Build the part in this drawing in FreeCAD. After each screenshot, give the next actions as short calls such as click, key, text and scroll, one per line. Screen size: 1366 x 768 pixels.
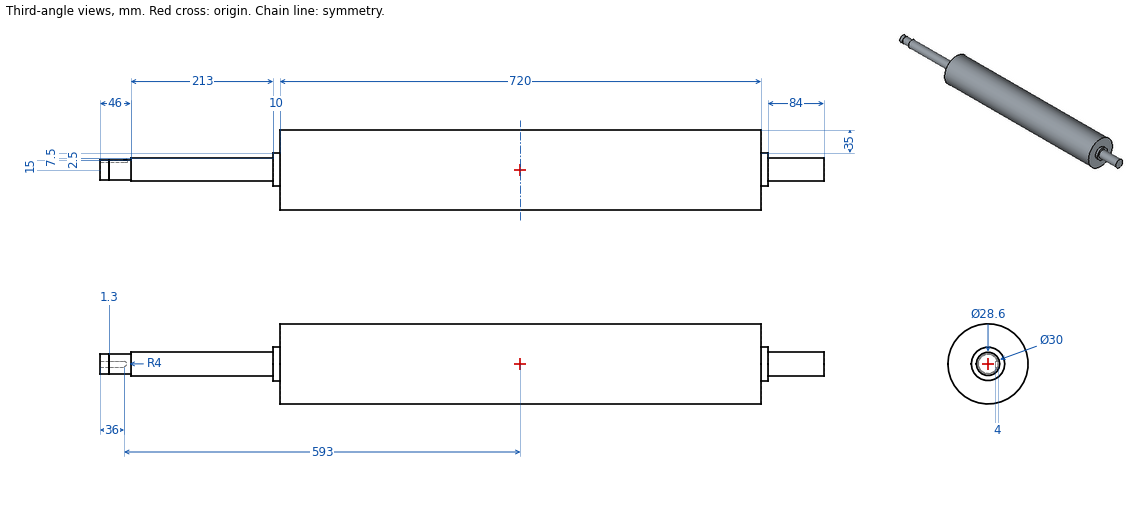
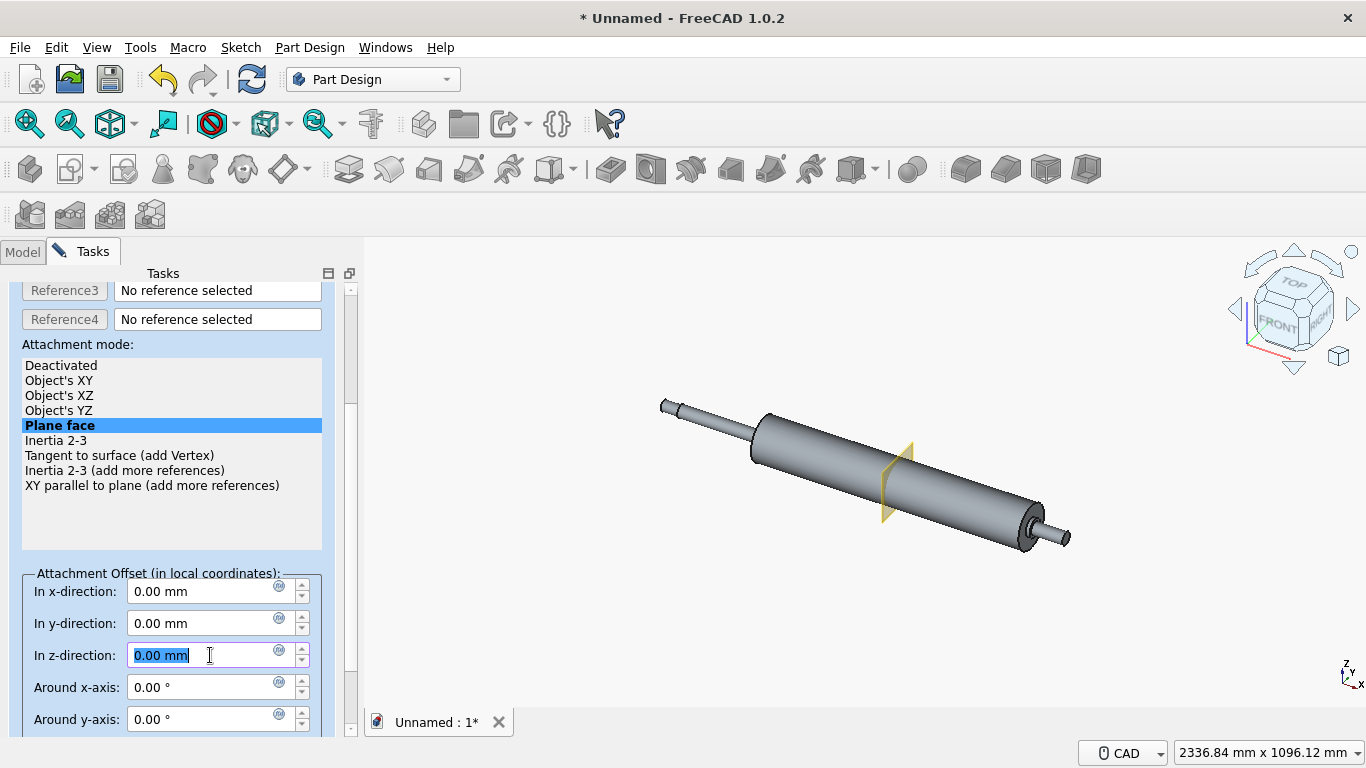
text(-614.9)
key(Tab)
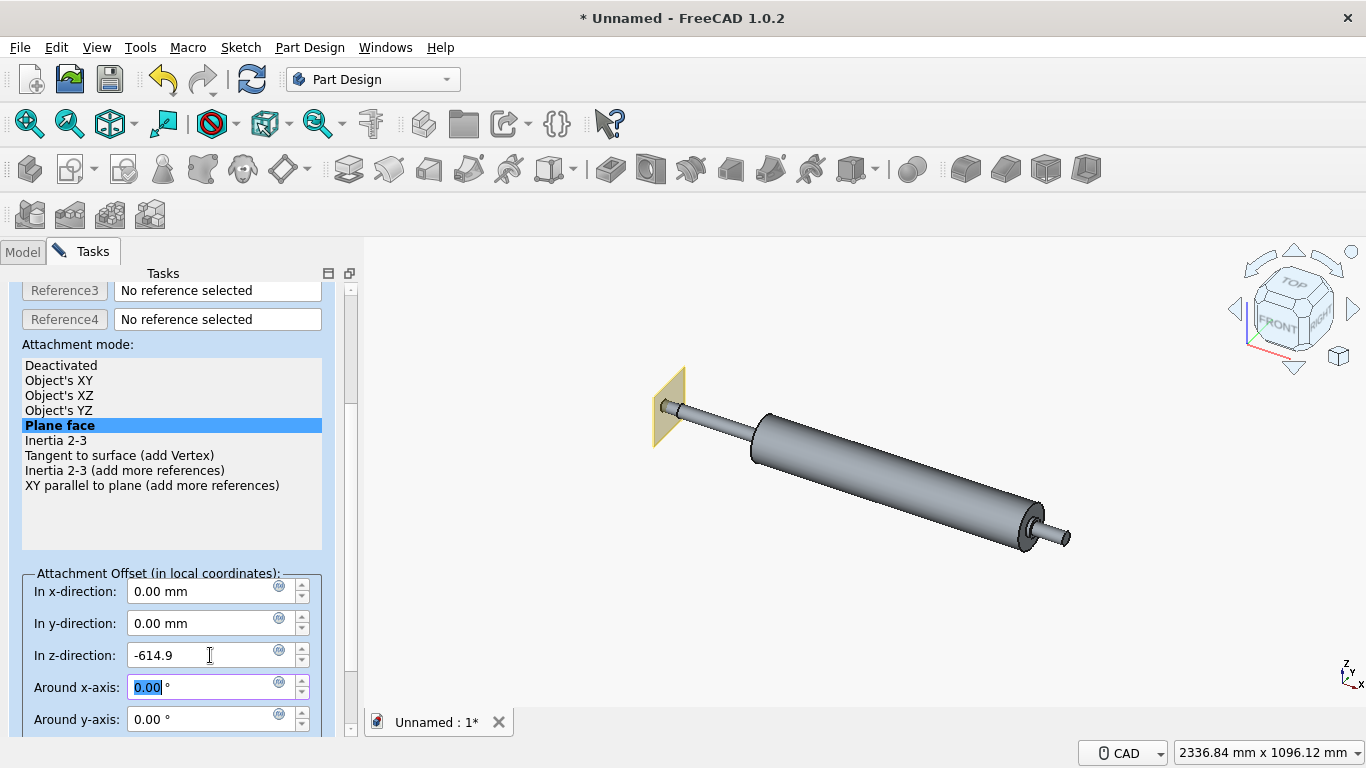
scroll(351, 510, up, 4)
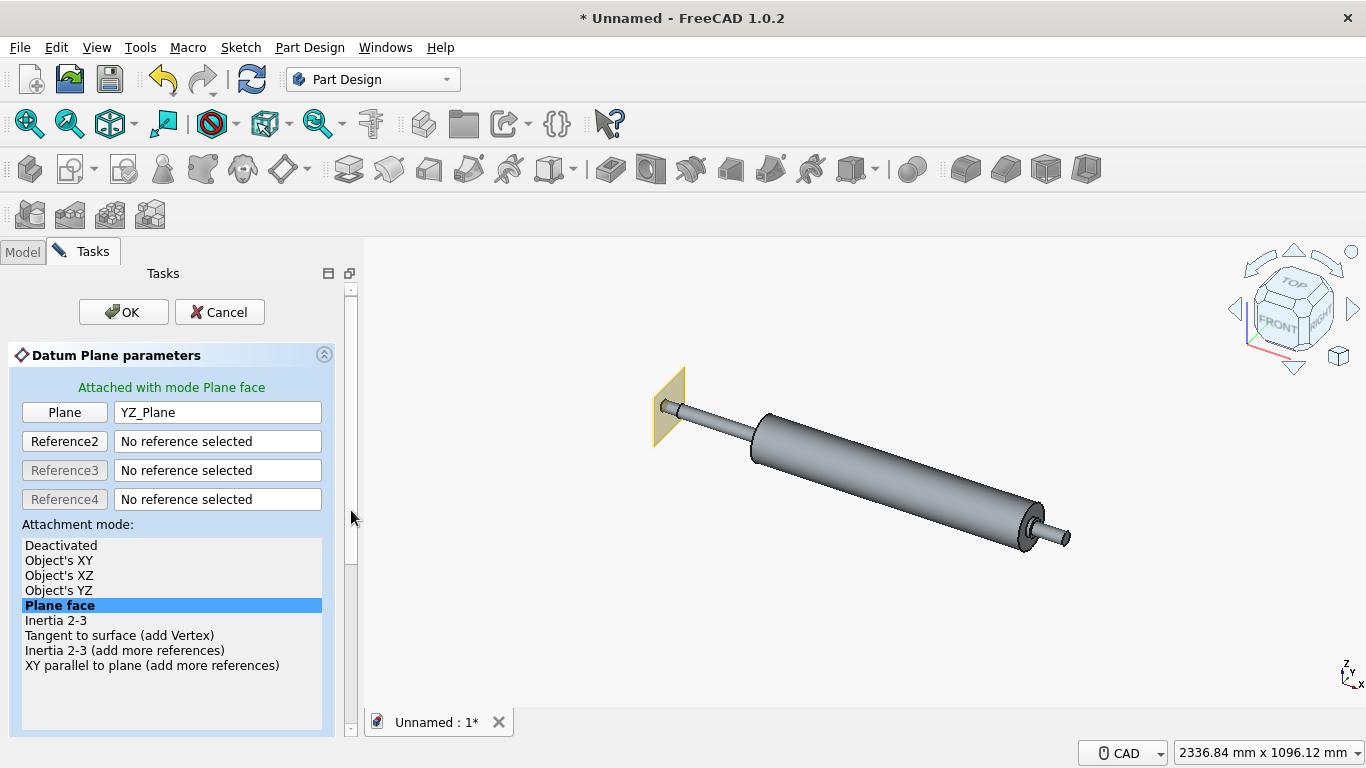
click(124, 312)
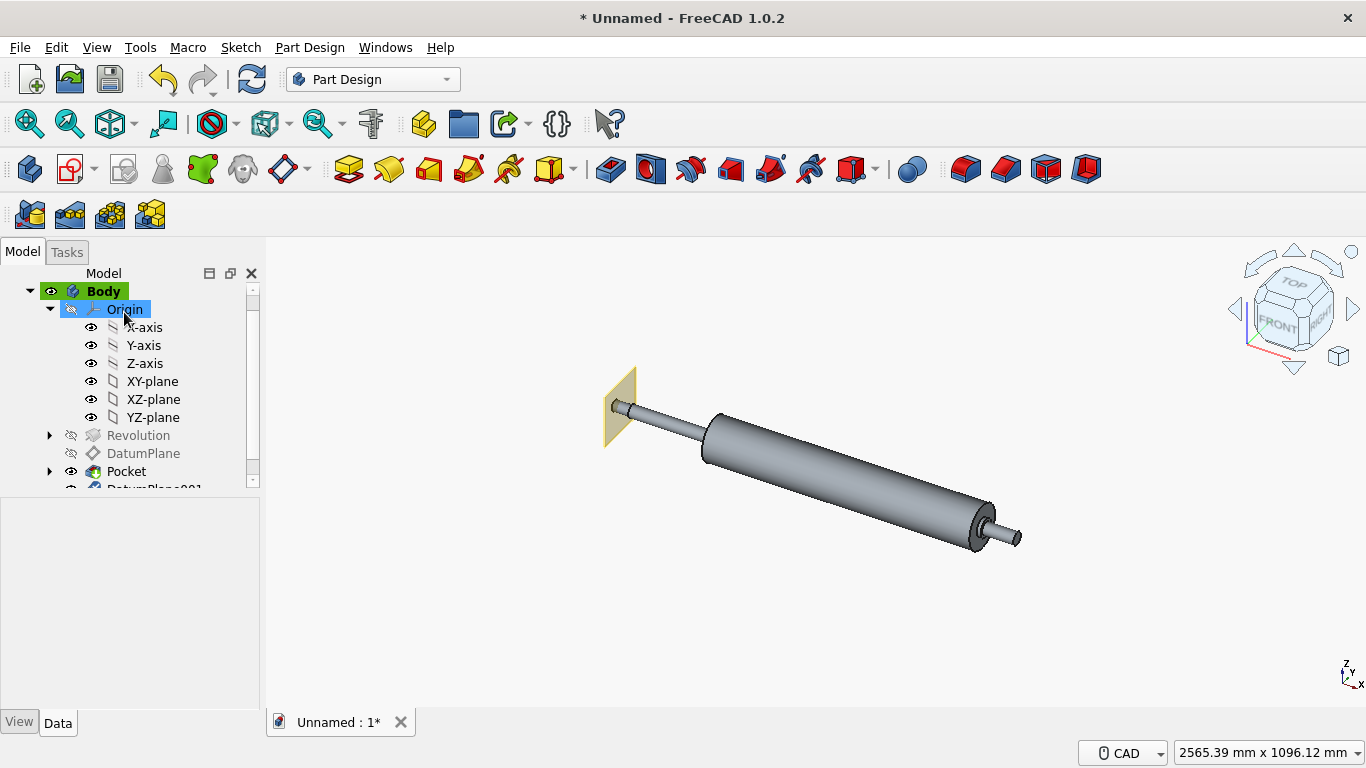
scroll(120, 377, down, 3)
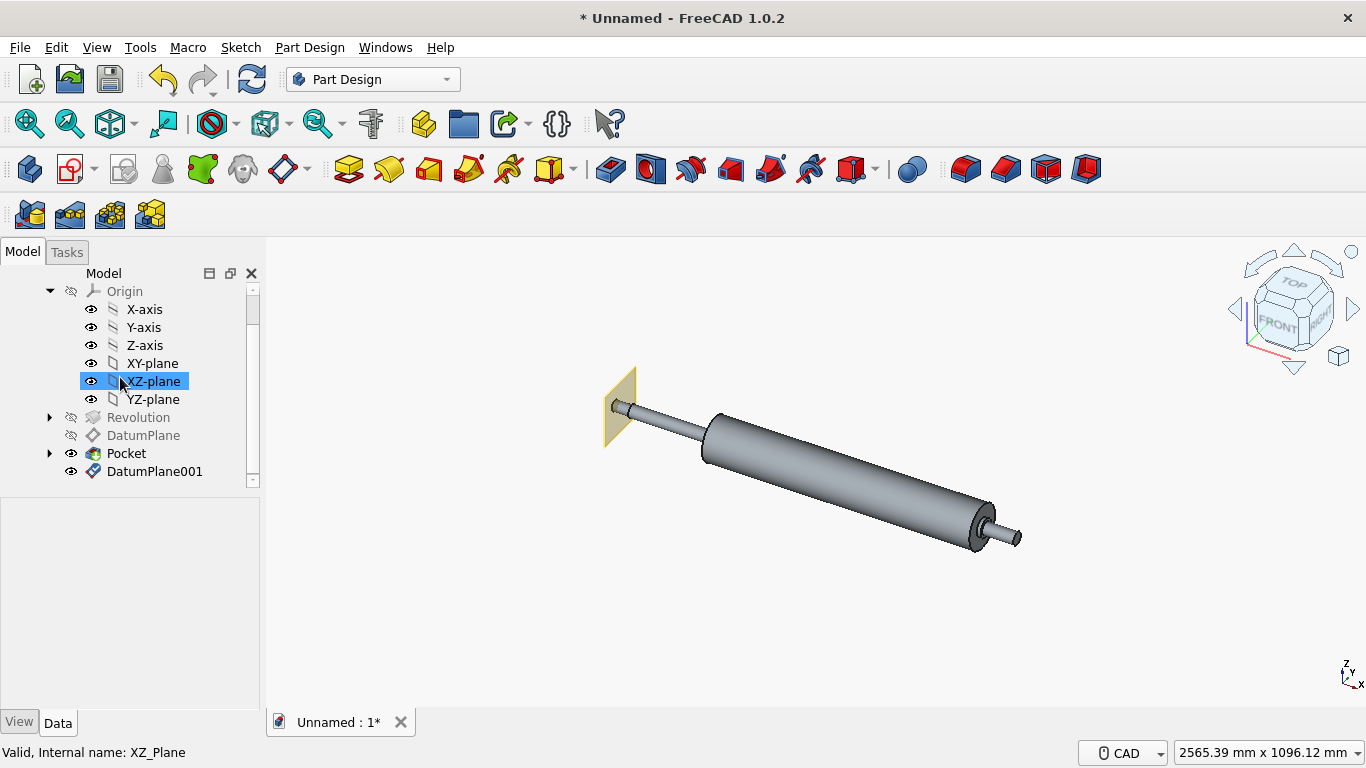
click(116, 471)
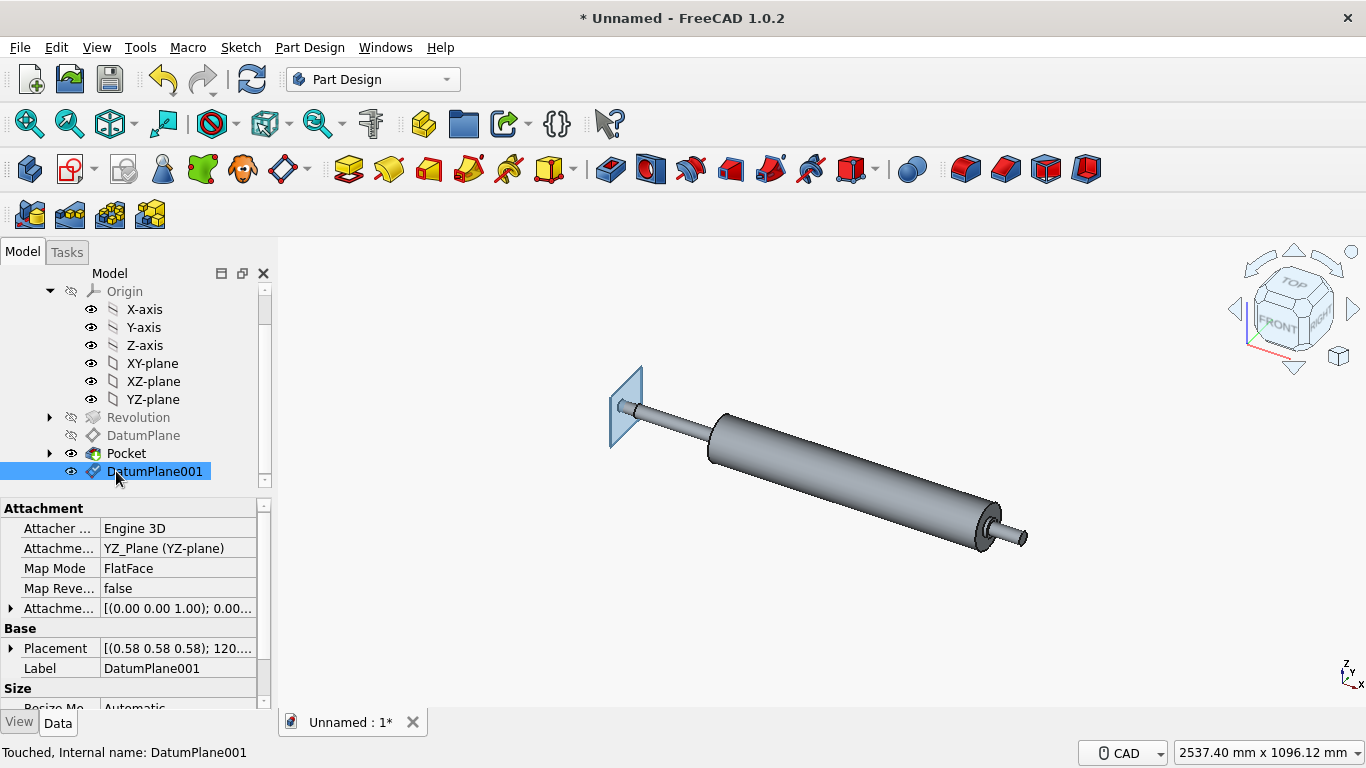
click(70, 170)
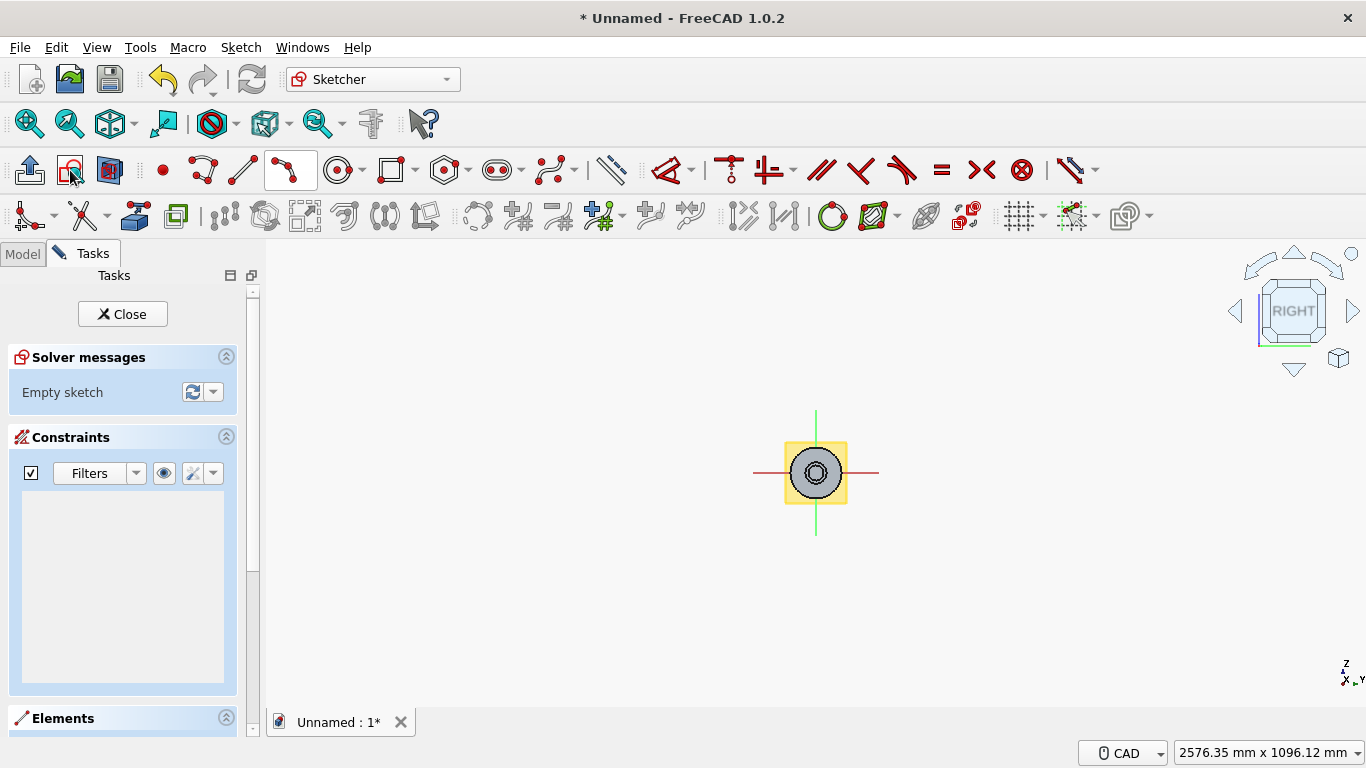
click(110, 170)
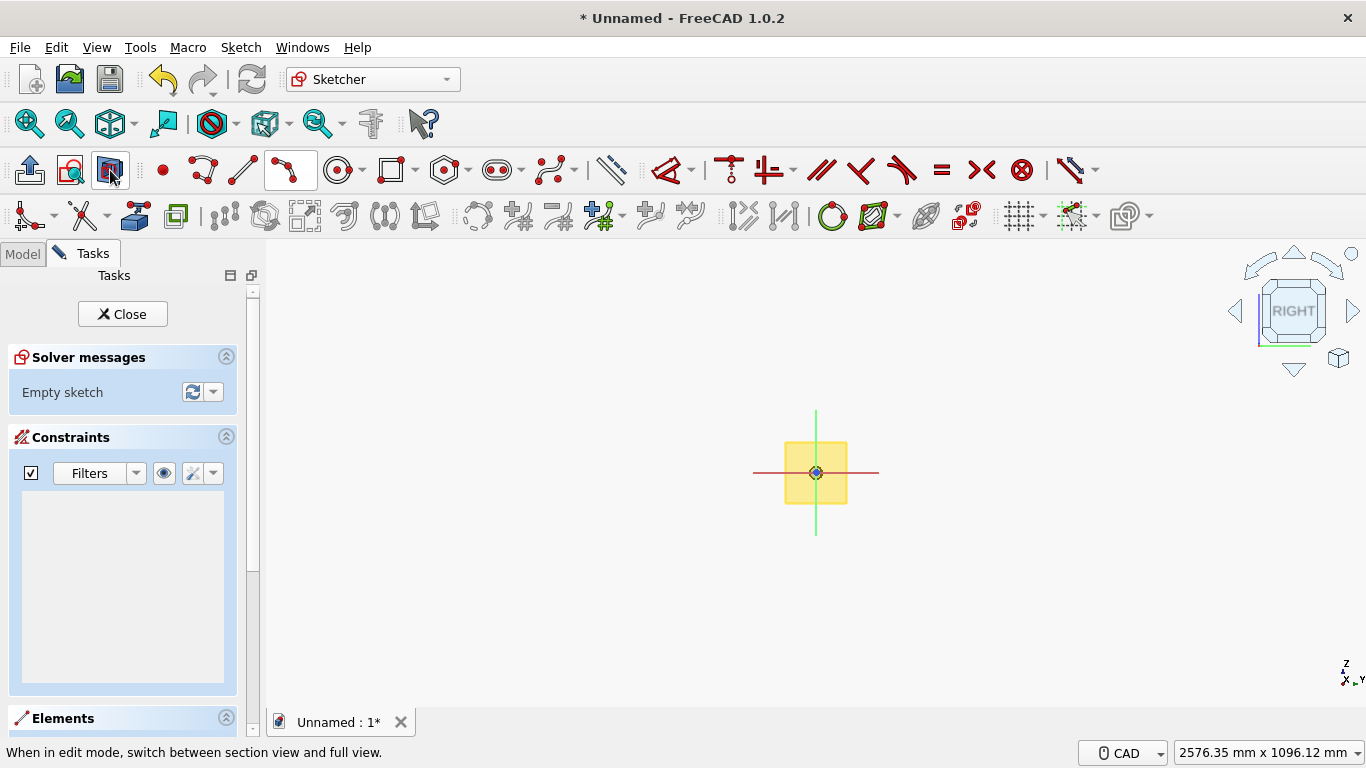
scroll(820, 473, up, 15)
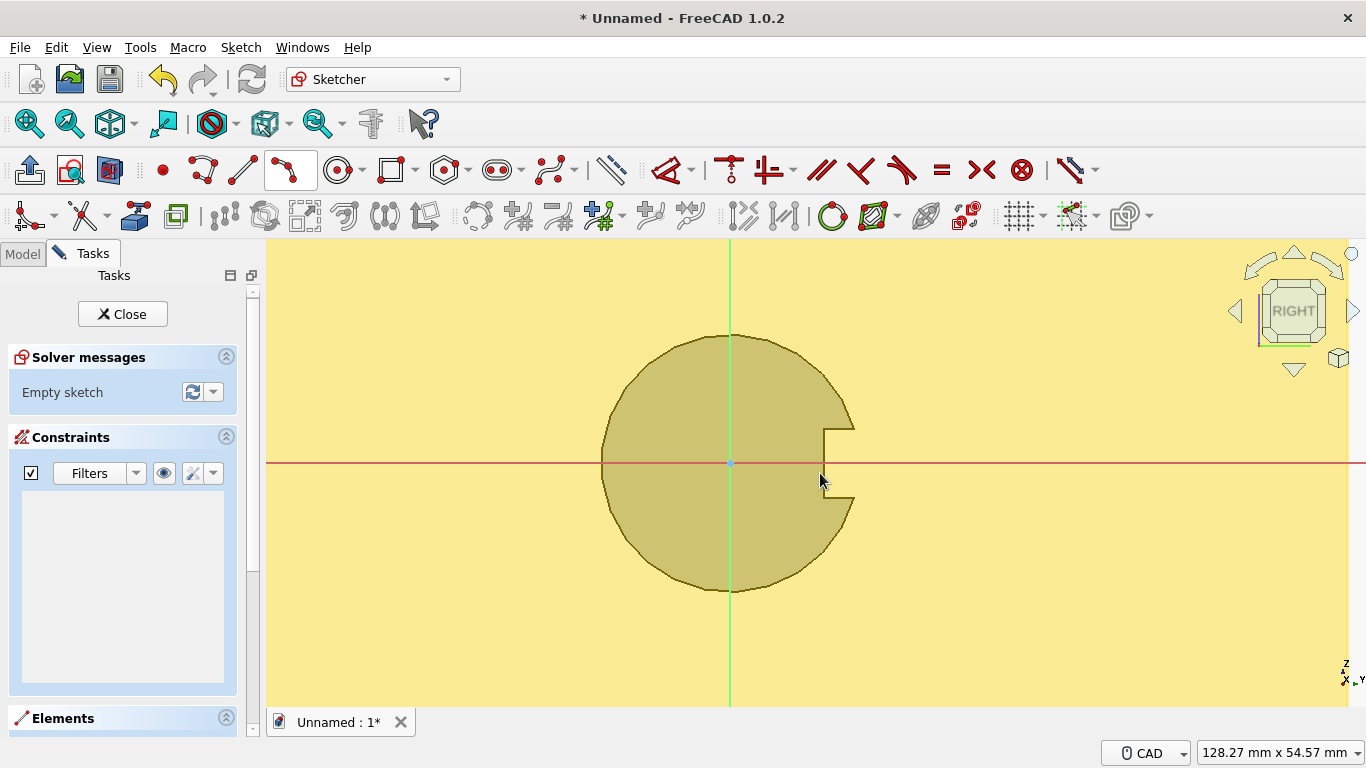
key(g)
key(c)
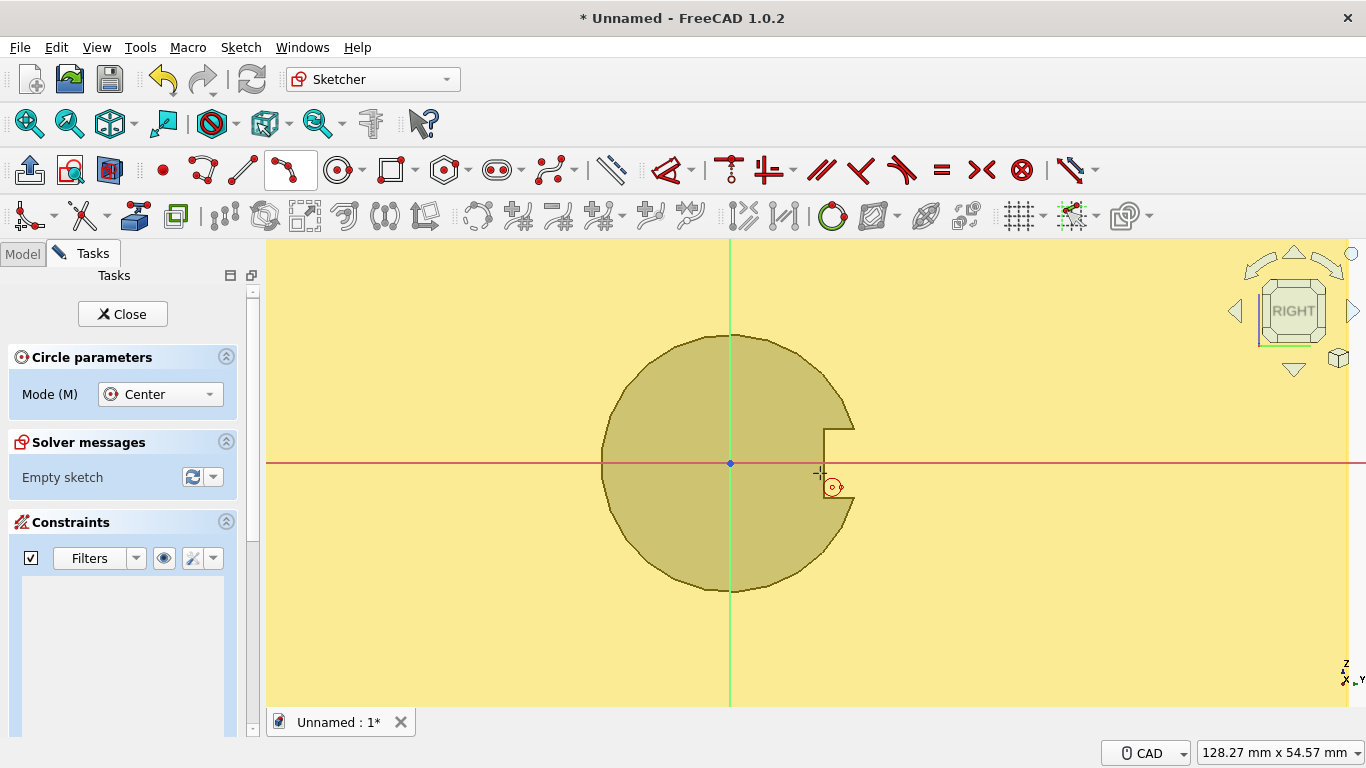
click(730, 463)
click(821, 372)